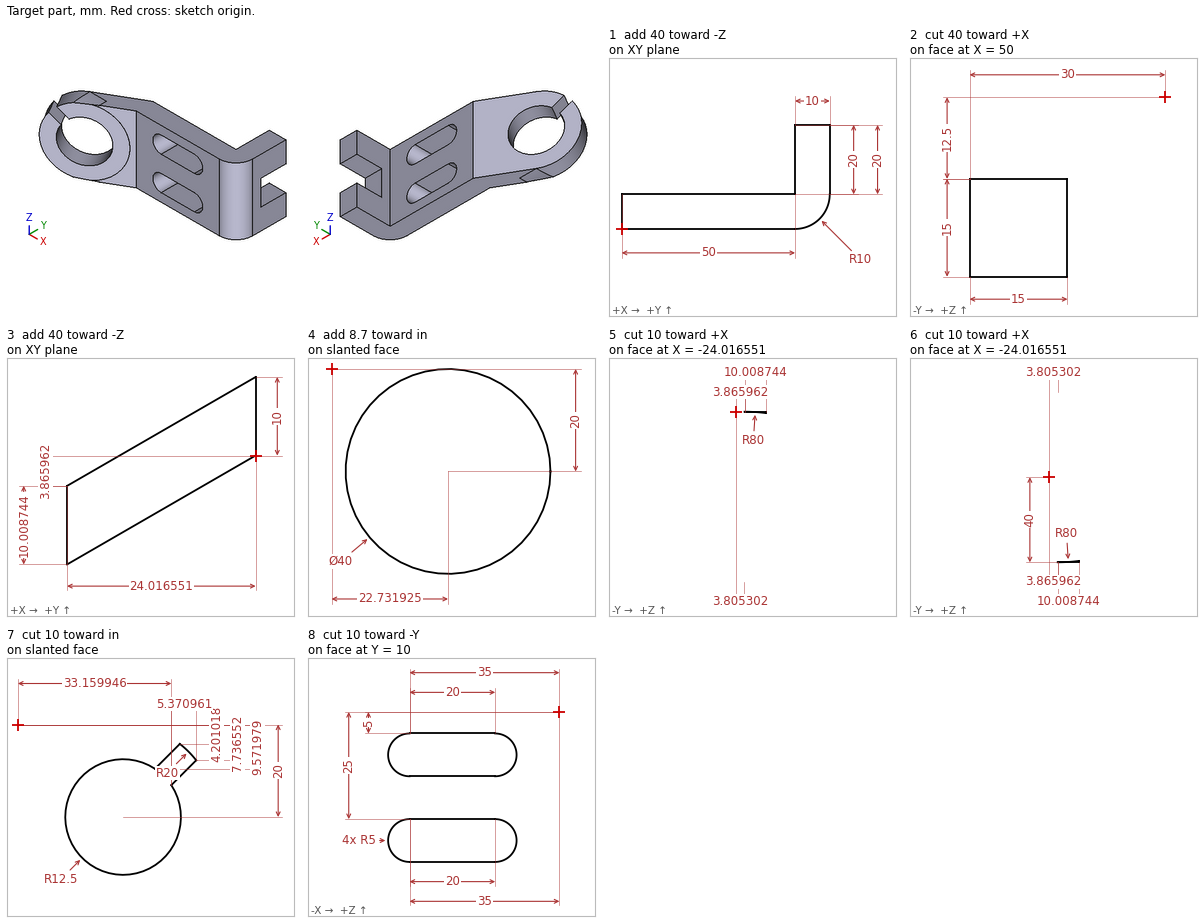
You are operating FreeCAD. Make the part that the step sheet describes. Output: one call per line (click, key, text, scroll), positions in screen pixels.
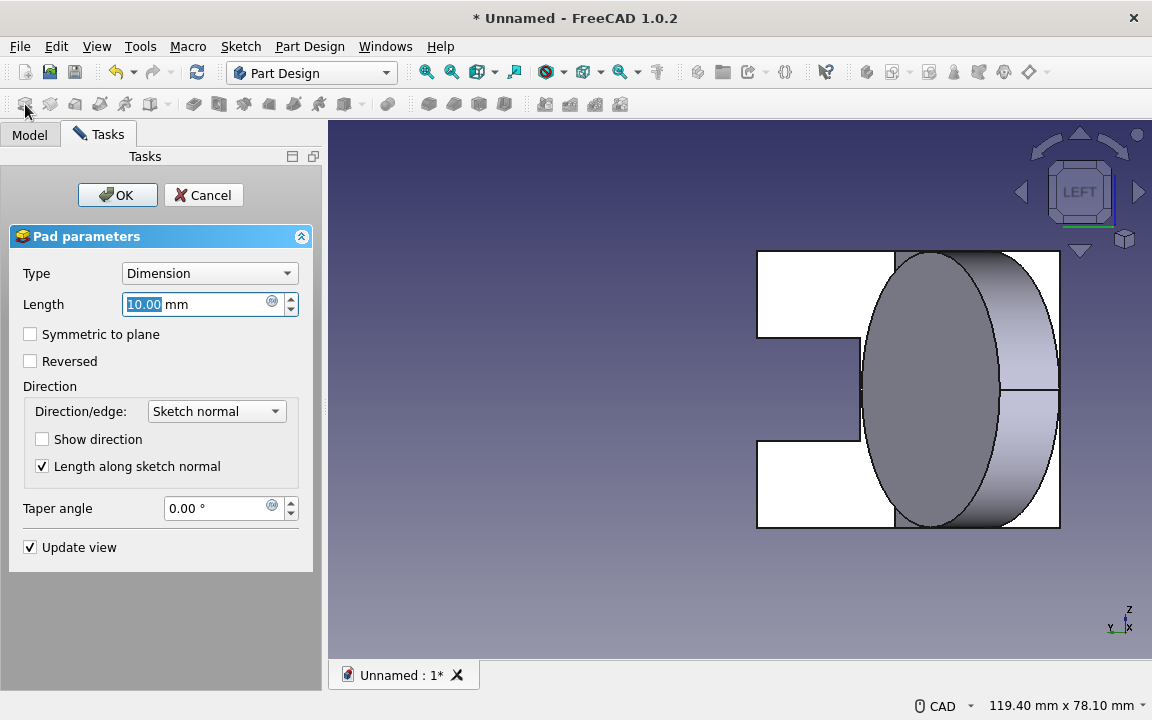
text(8.7)
key(Tab)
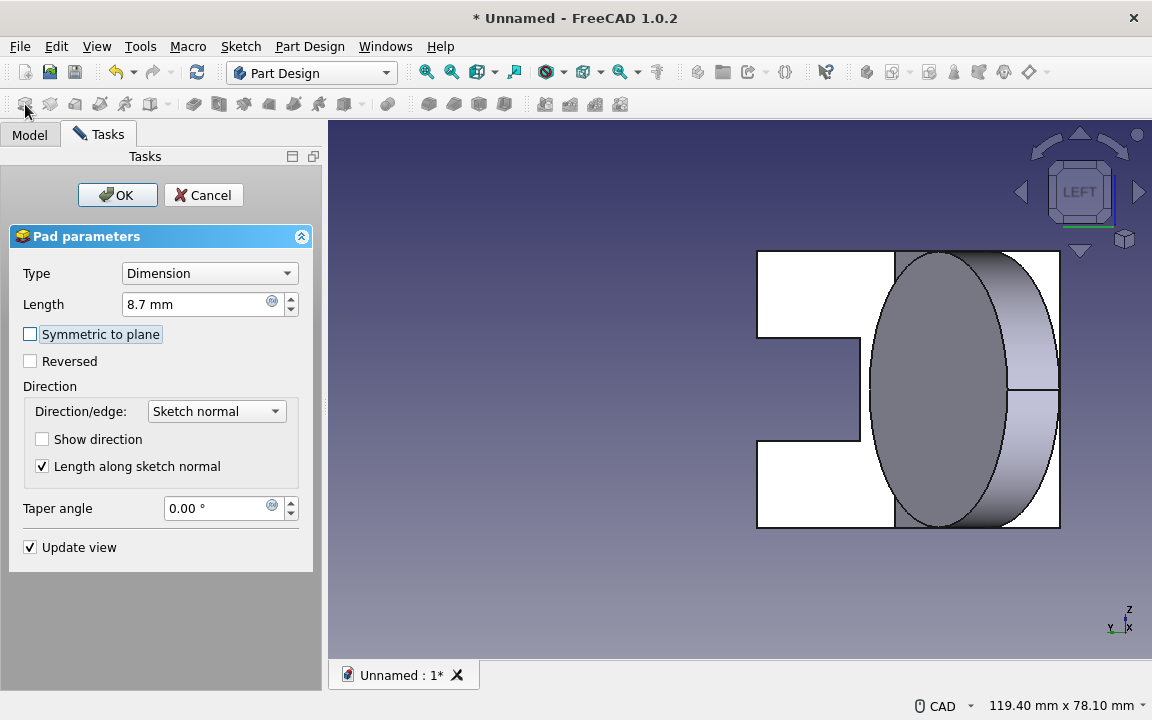
click(31, 361)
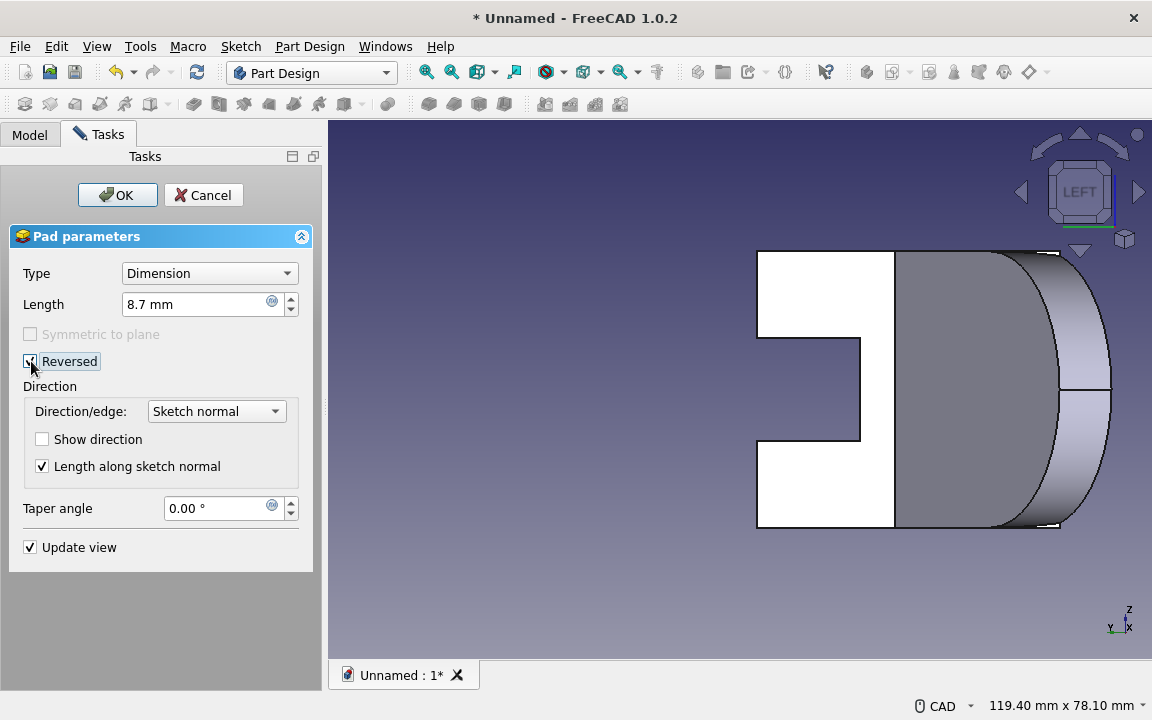
click(118, 195)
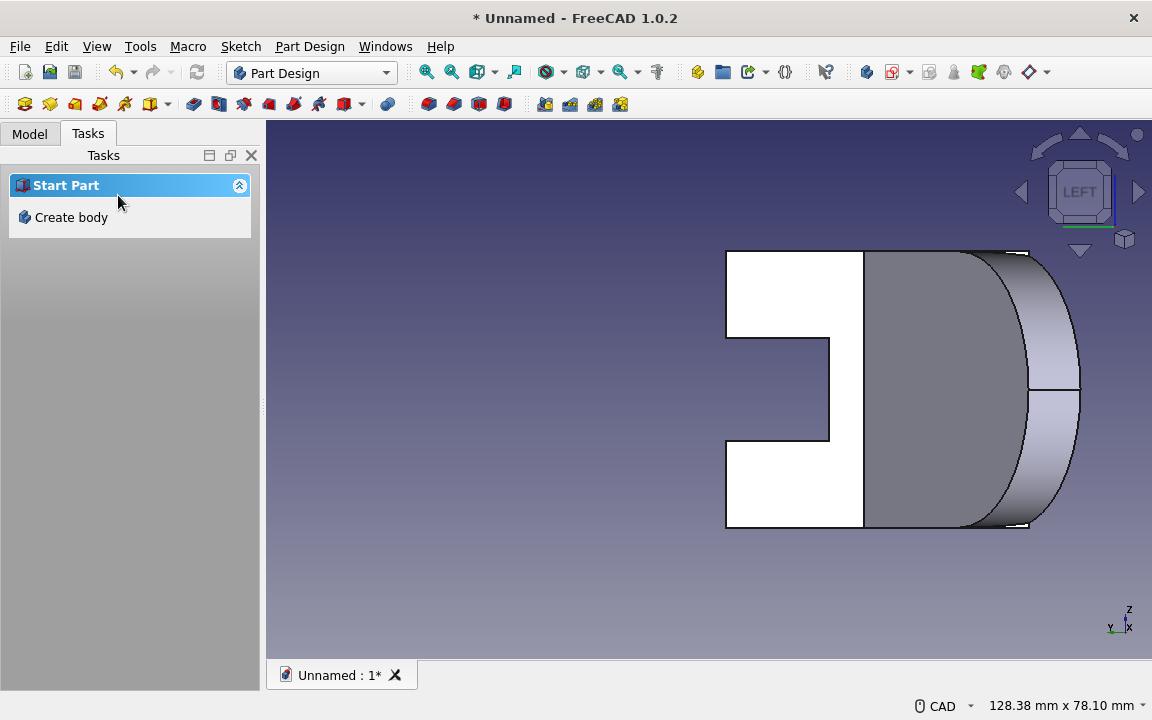
key(2)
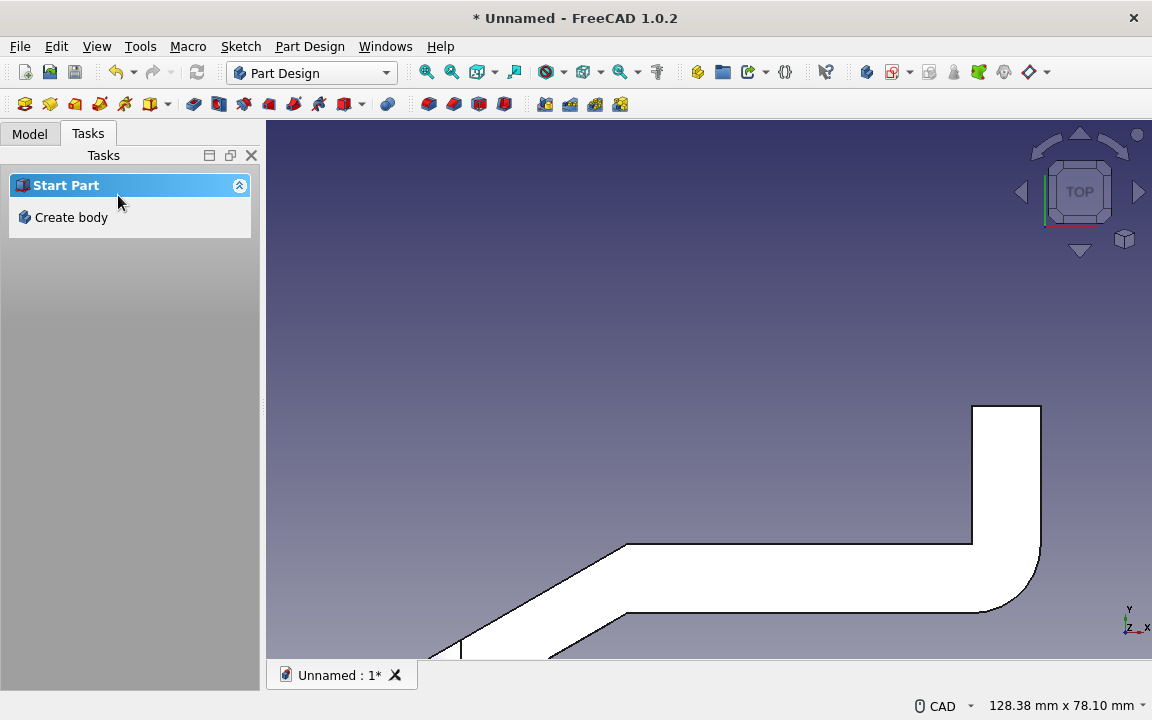
click(427, 72)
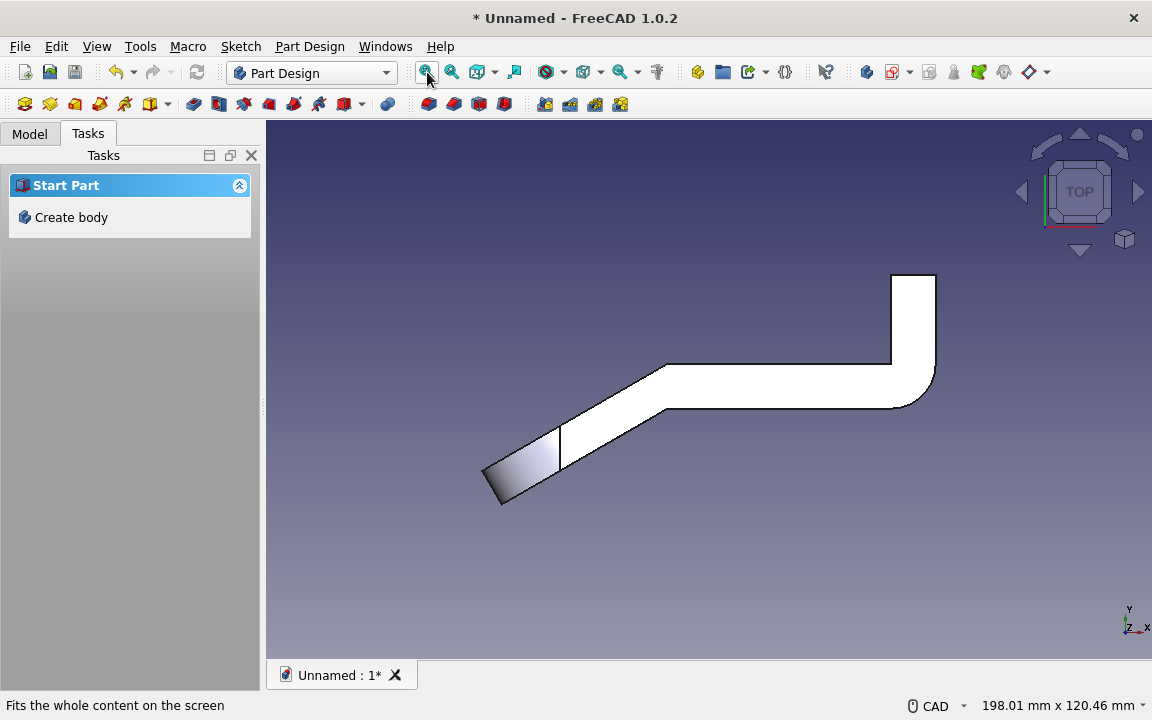
key(6)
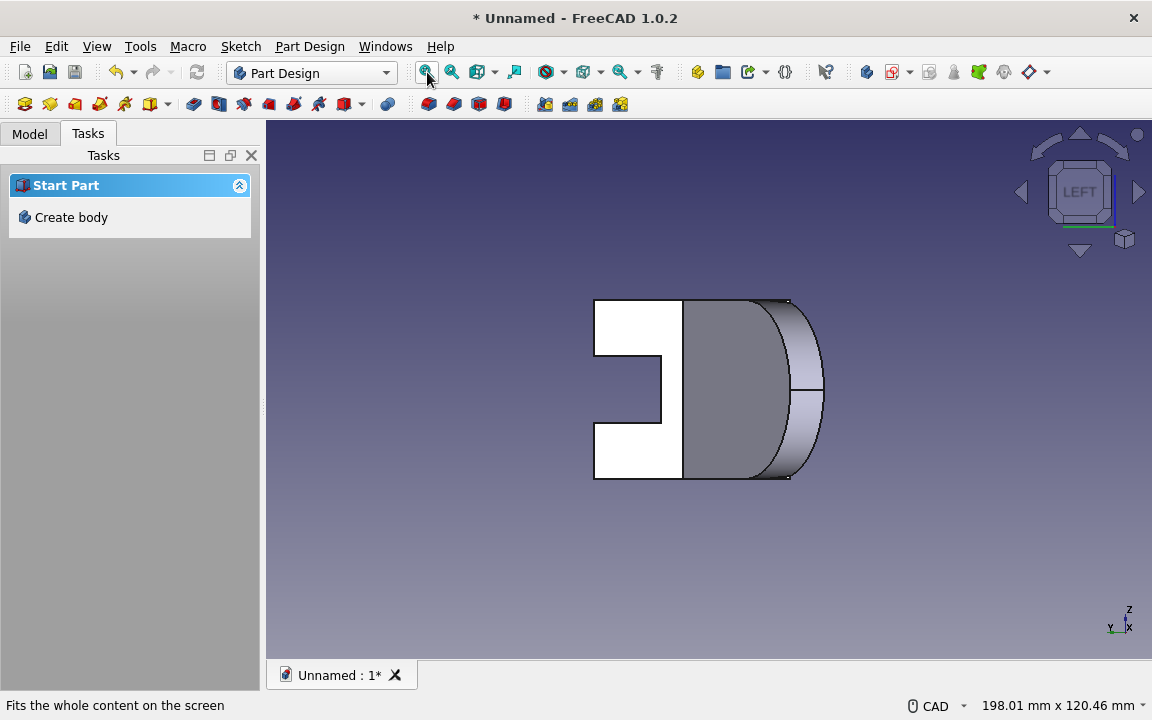
click(427, 72)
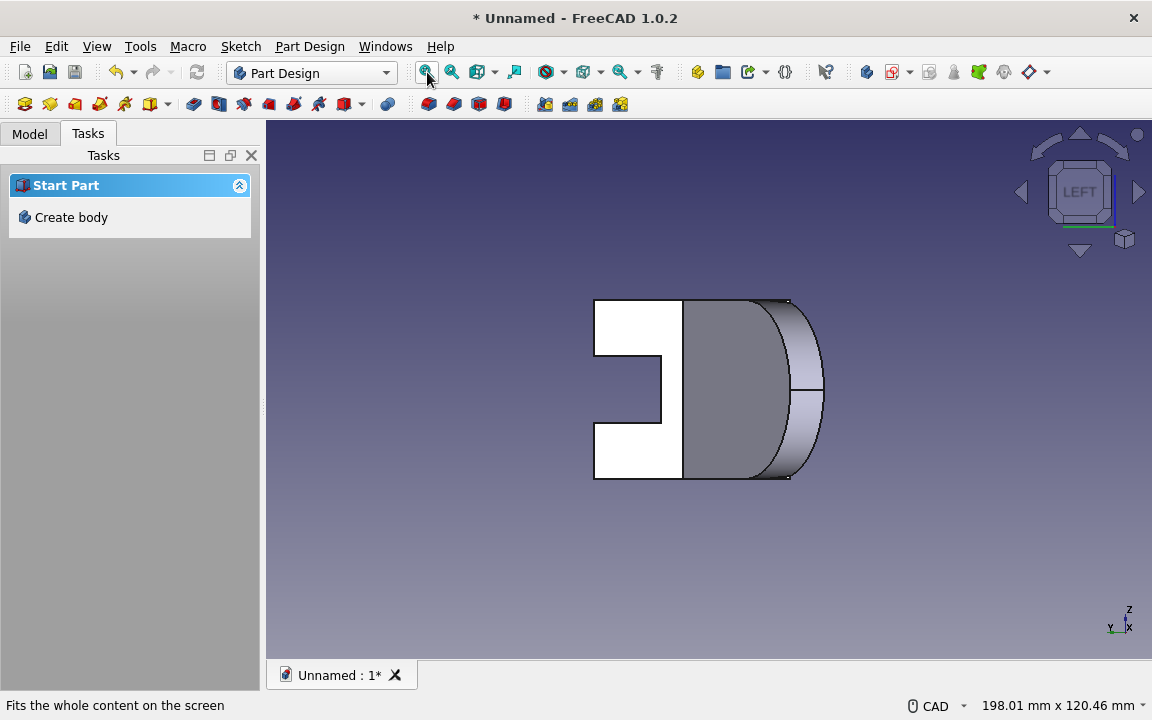
scroll(787, 300, up, 13)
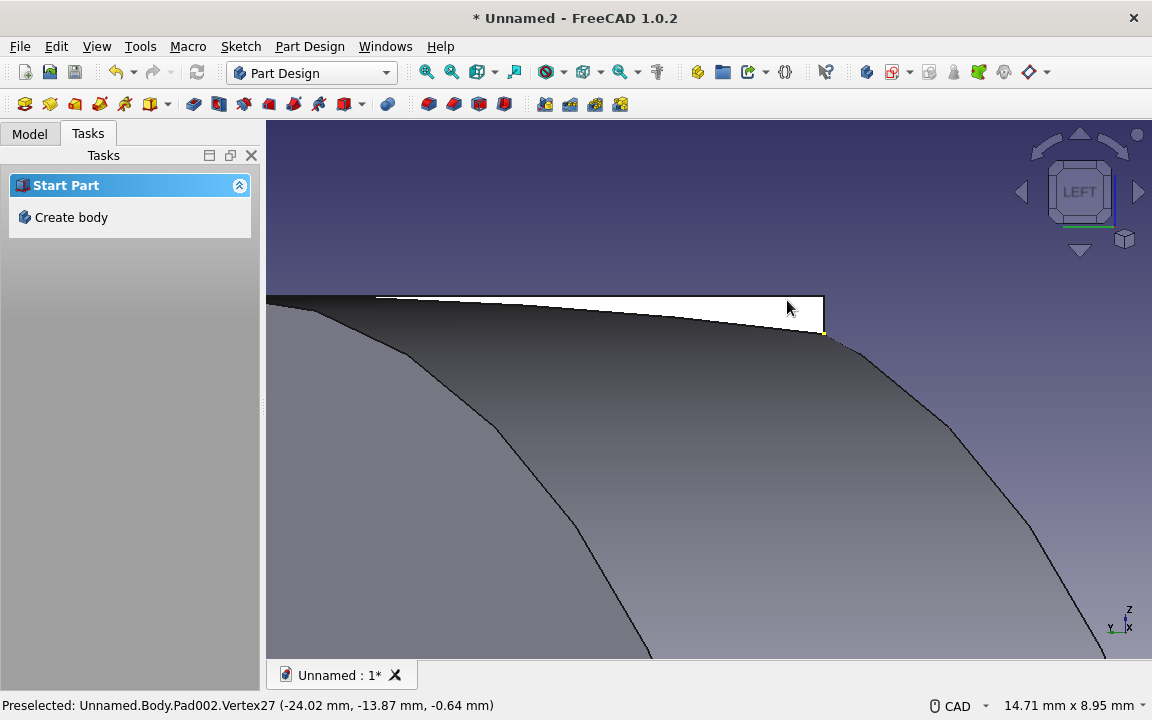
click(781, 314)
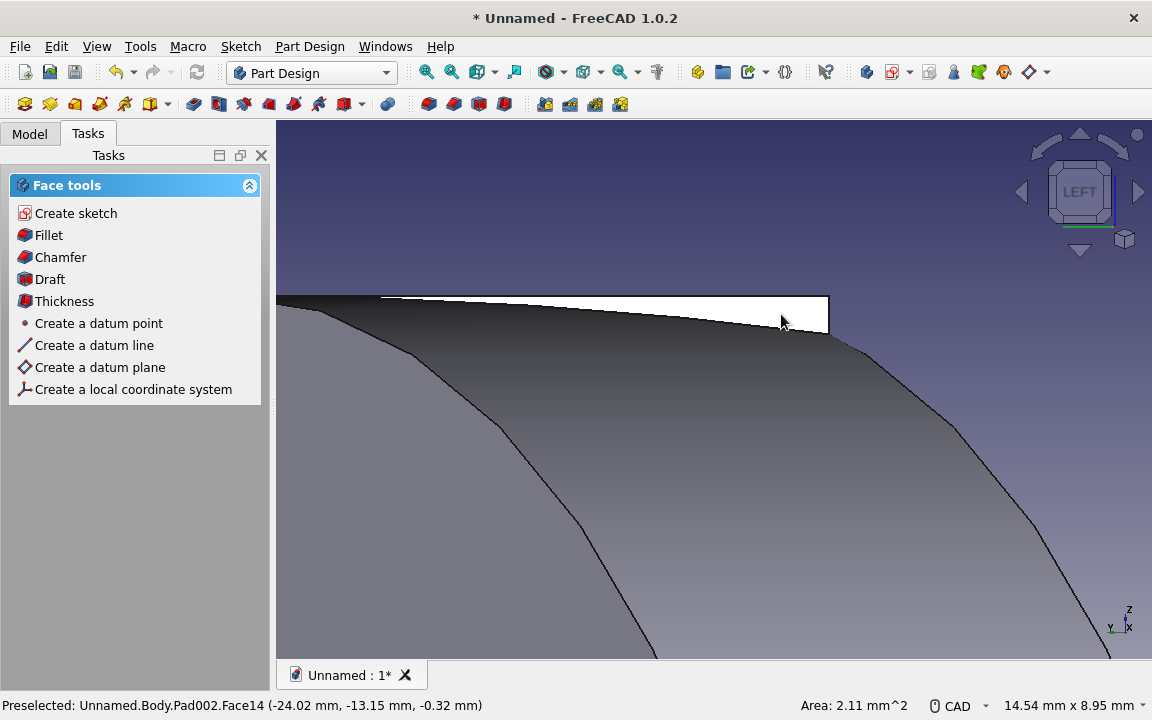
click(892, 72)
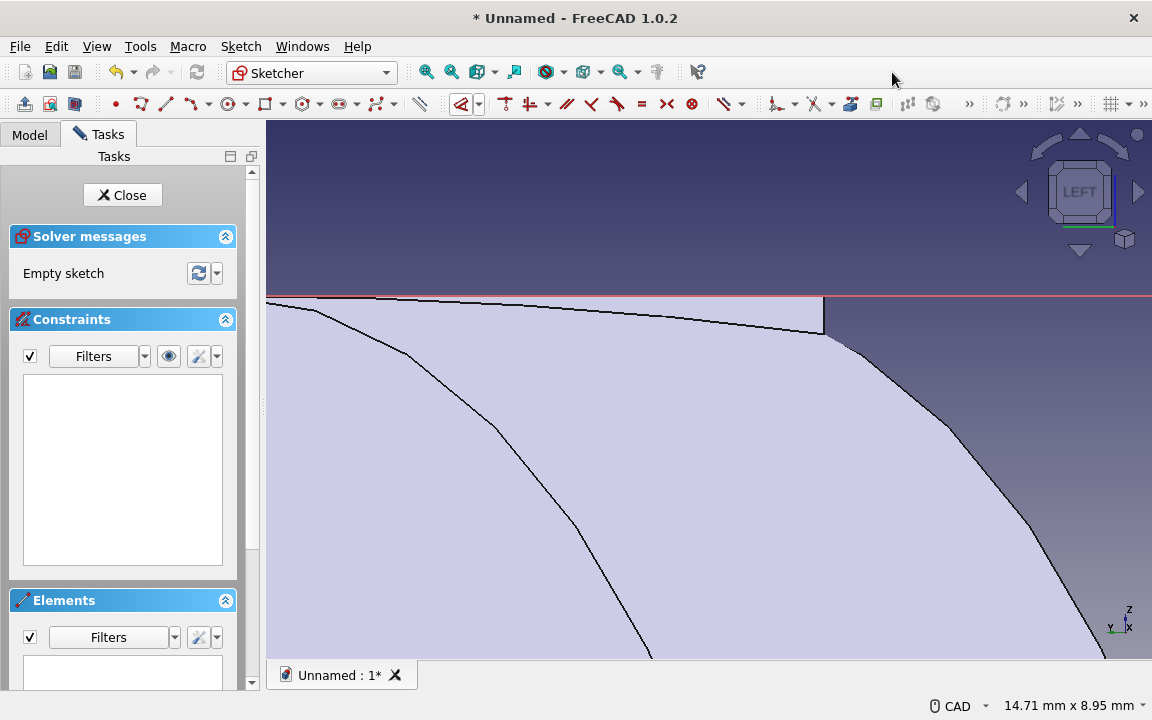
click(75, 104)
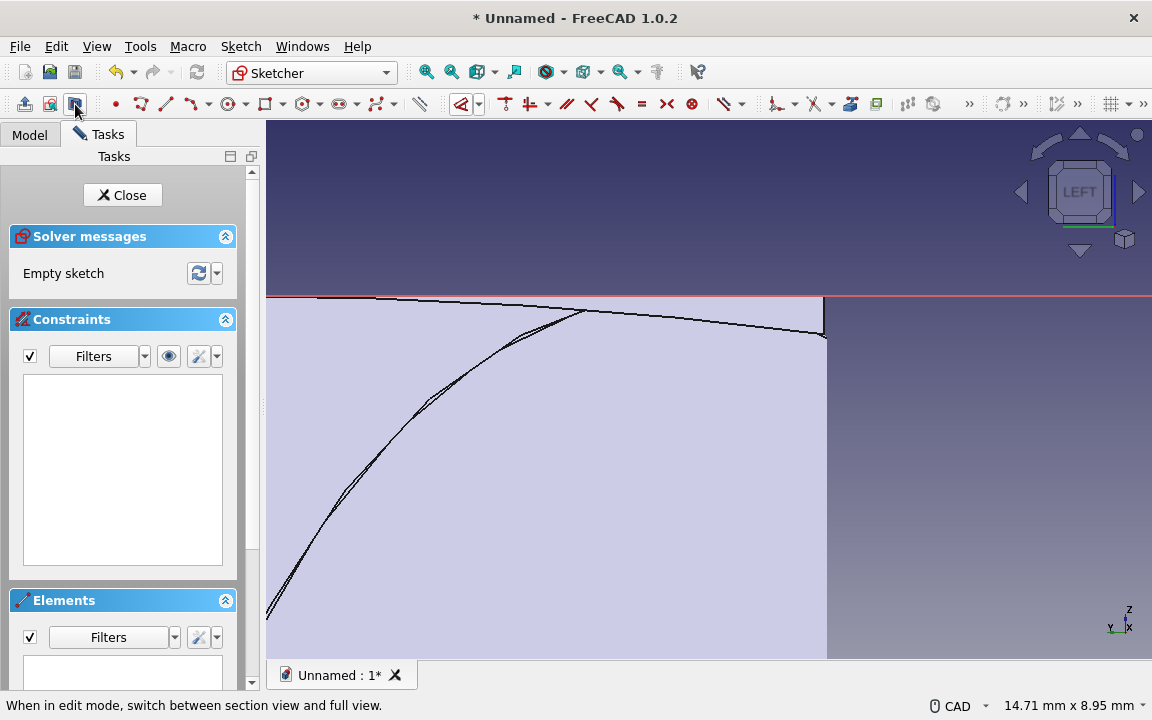
scroll(925, 480, down, 3)